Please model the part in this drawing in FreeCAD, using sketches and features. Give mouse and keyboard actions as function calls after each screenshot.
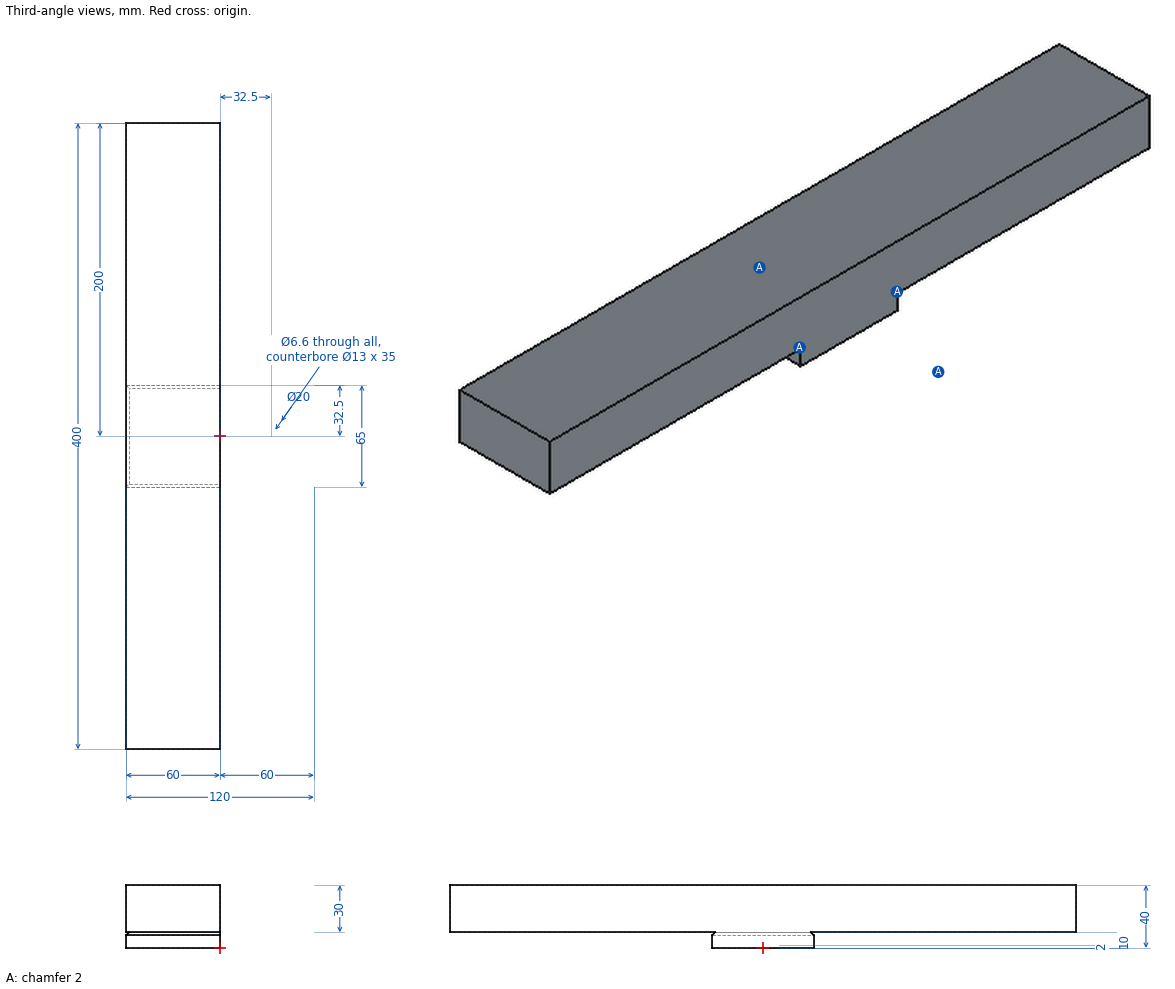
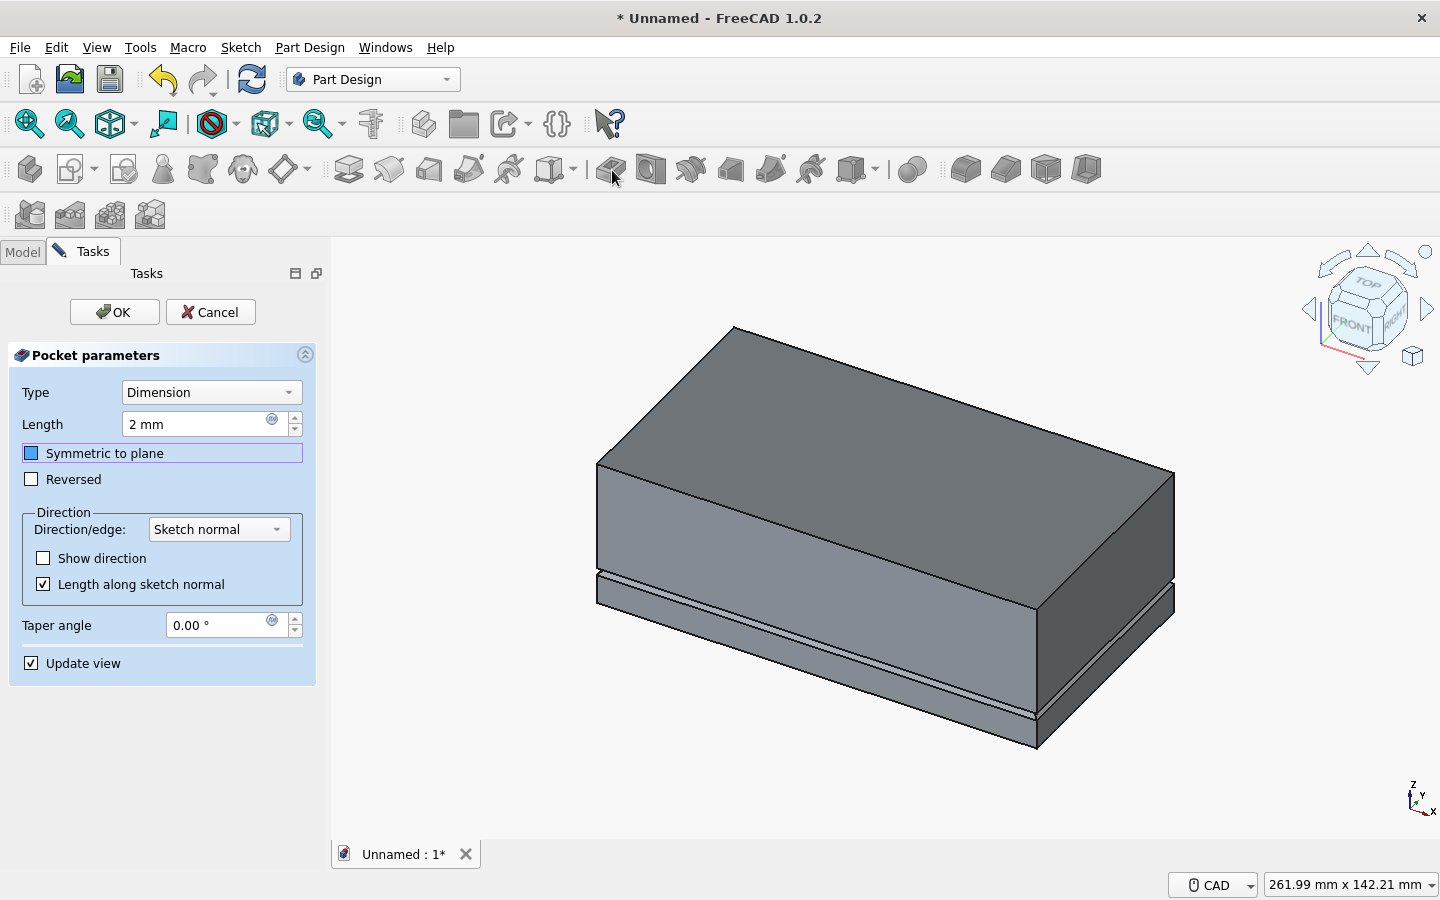
click(30, 479)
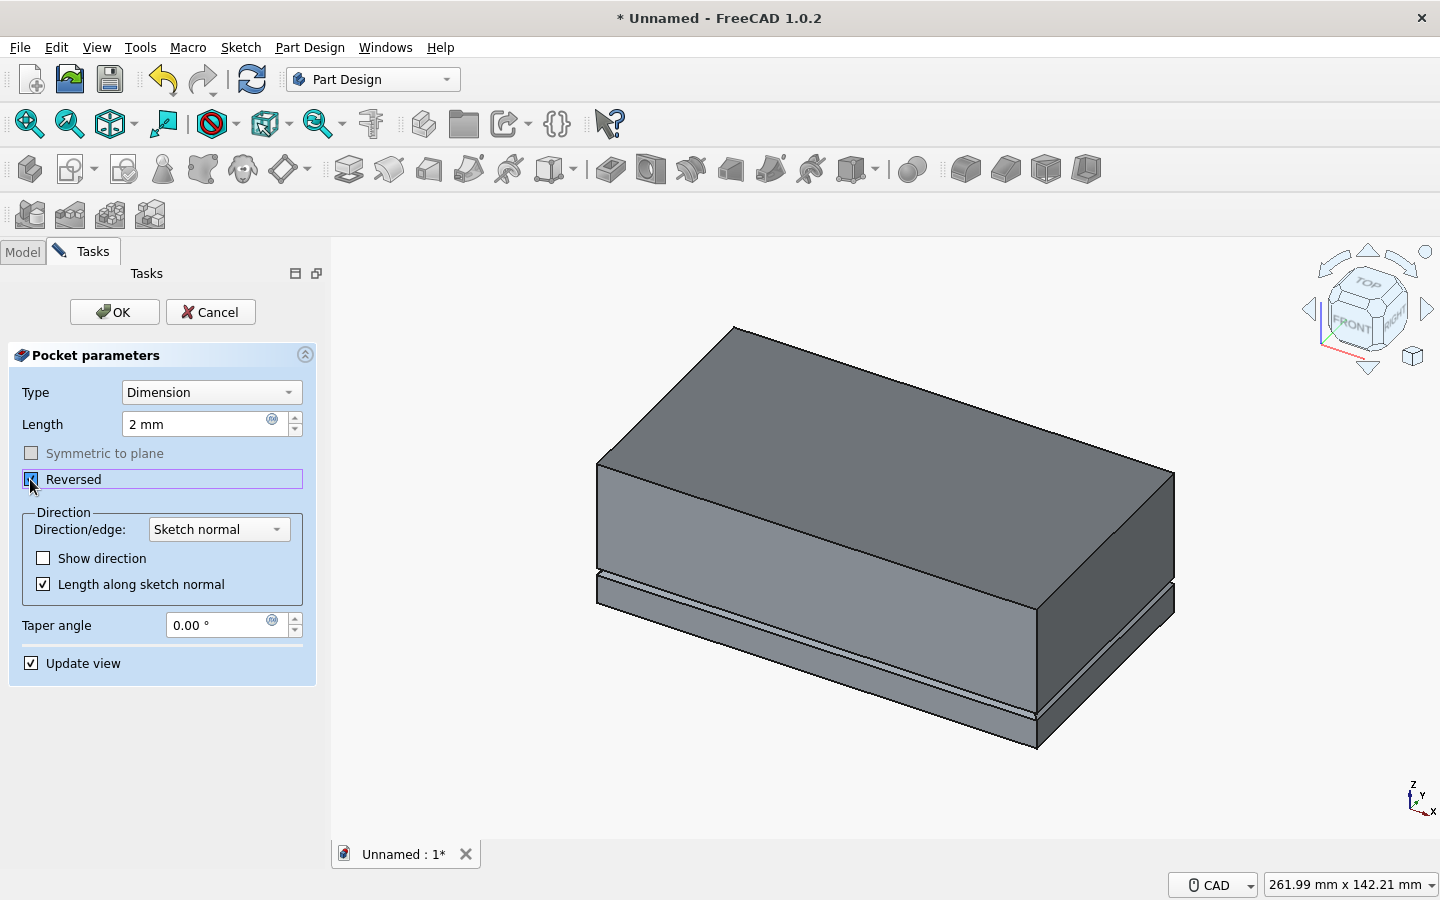
click(115, 312)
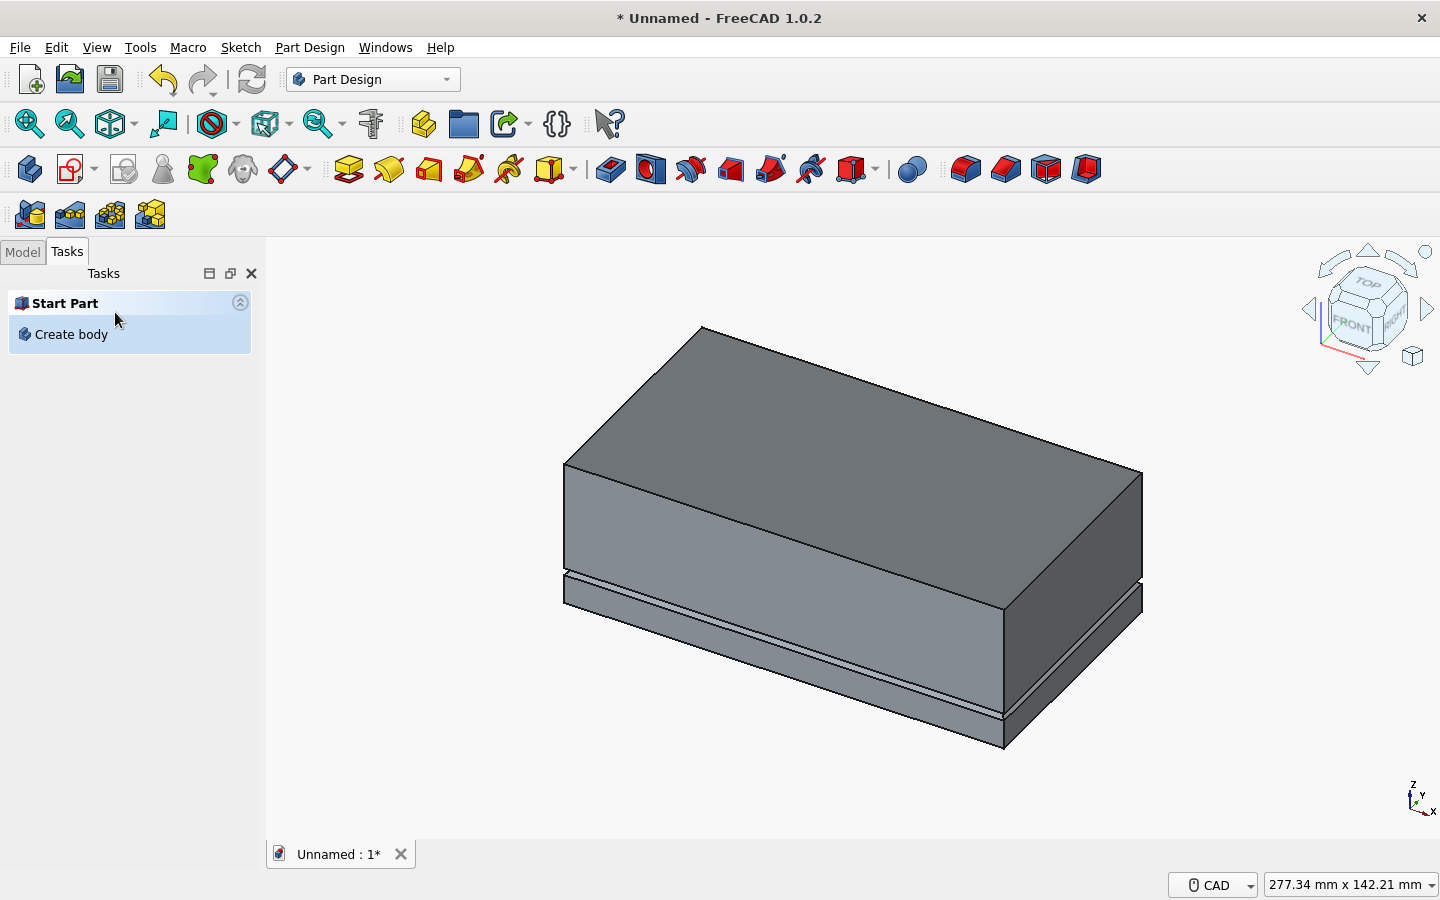
click(916, 488)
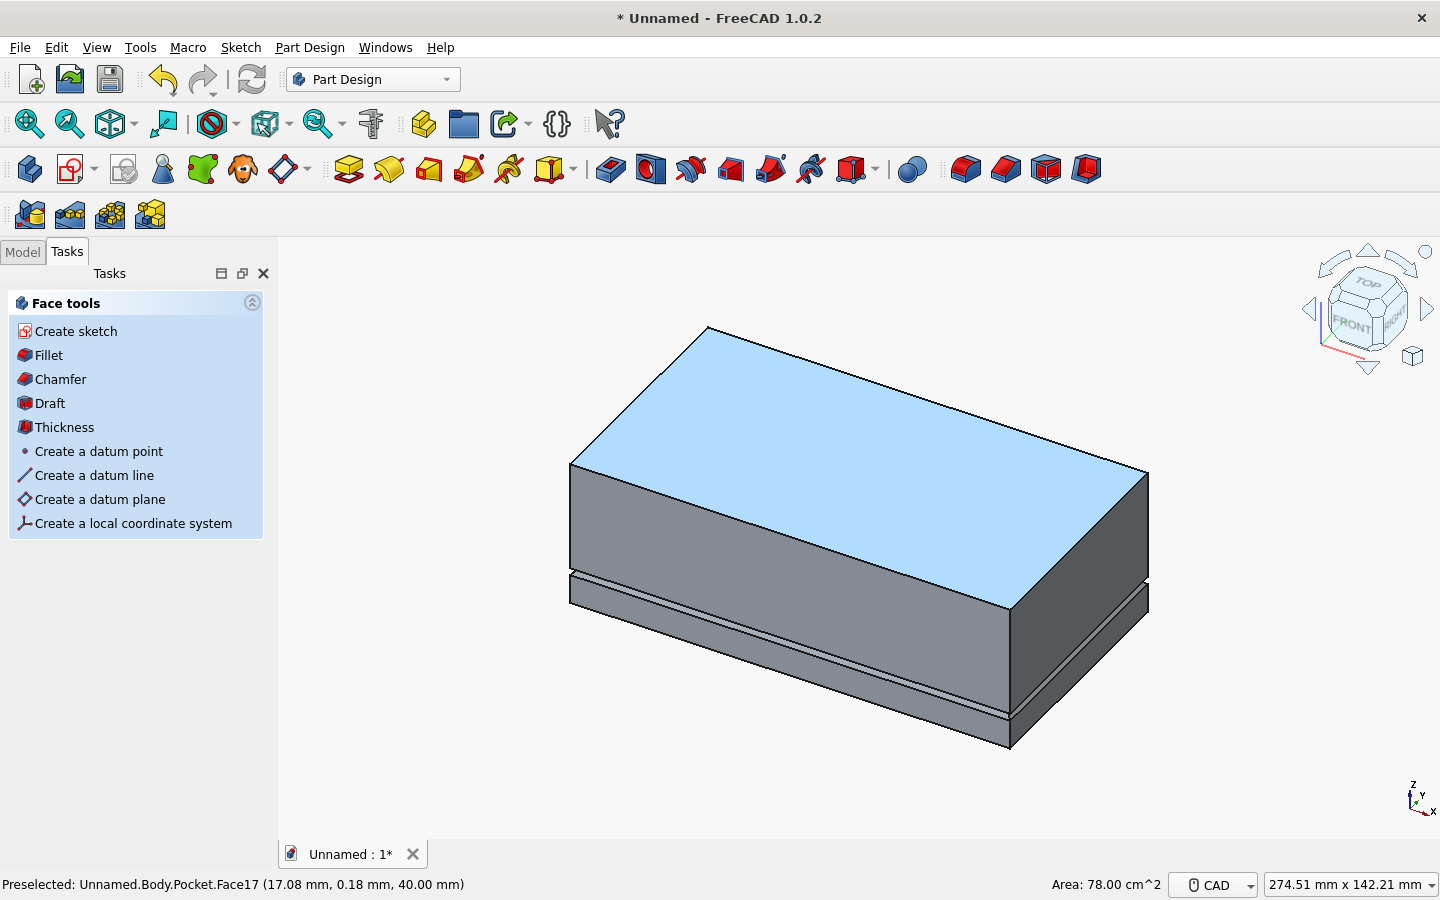
click(70, 170)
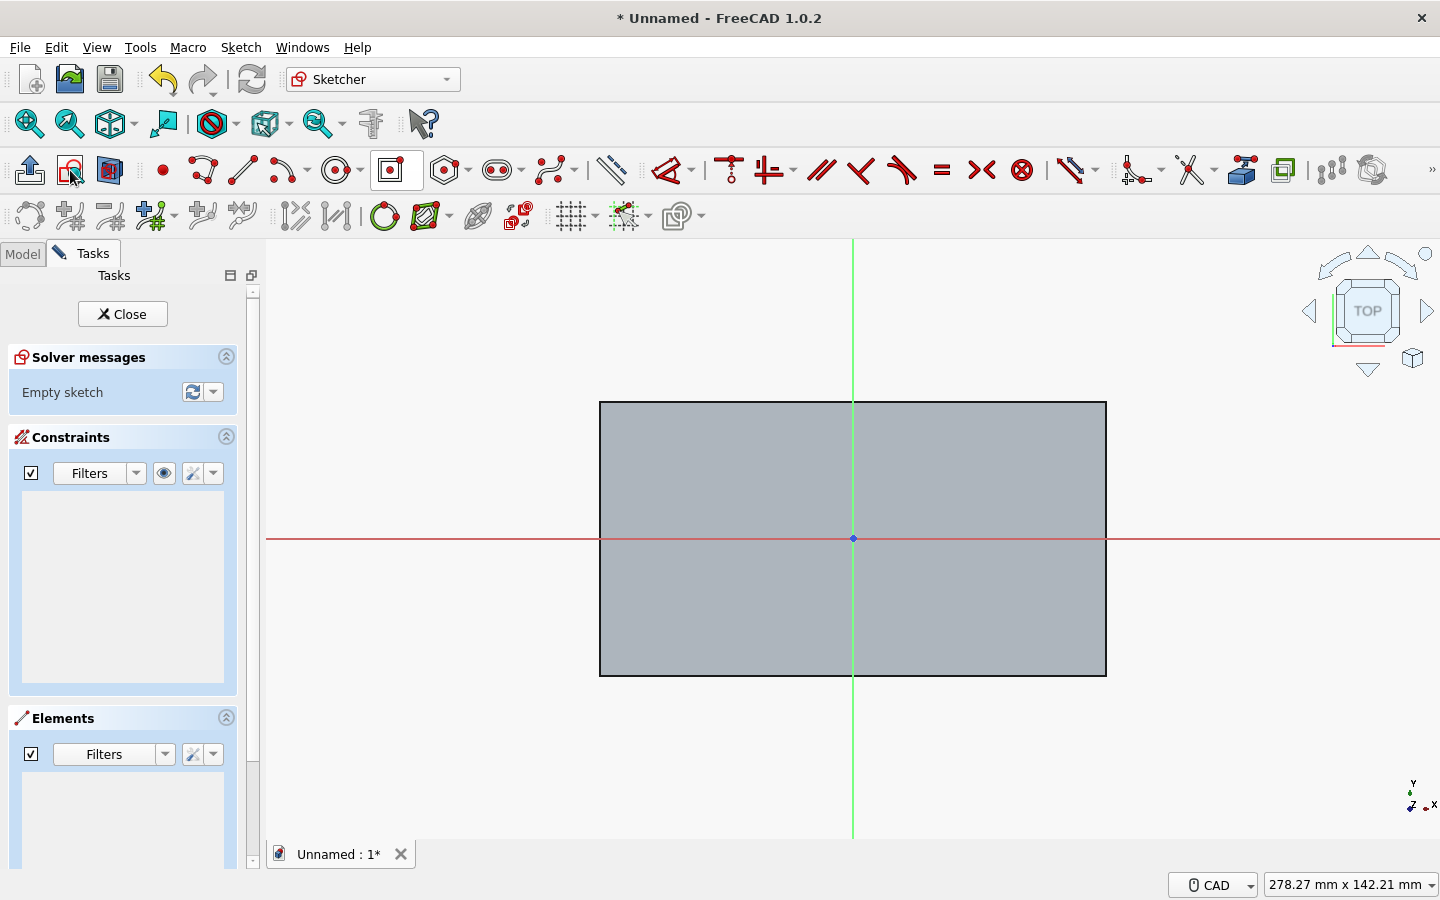
scroll(1007, 539, up, 13)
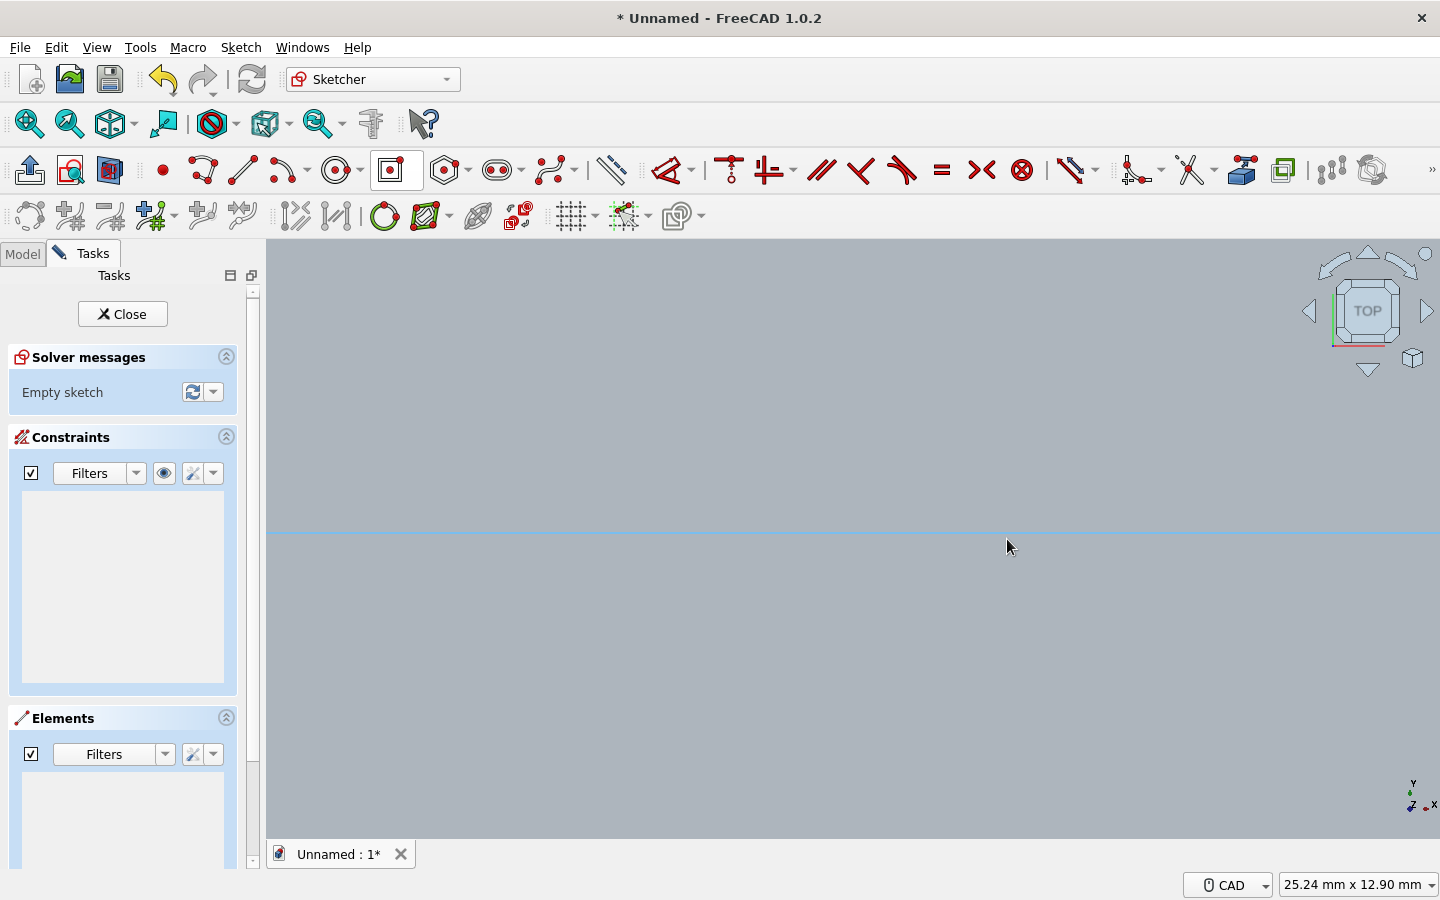
key(g)
key(c)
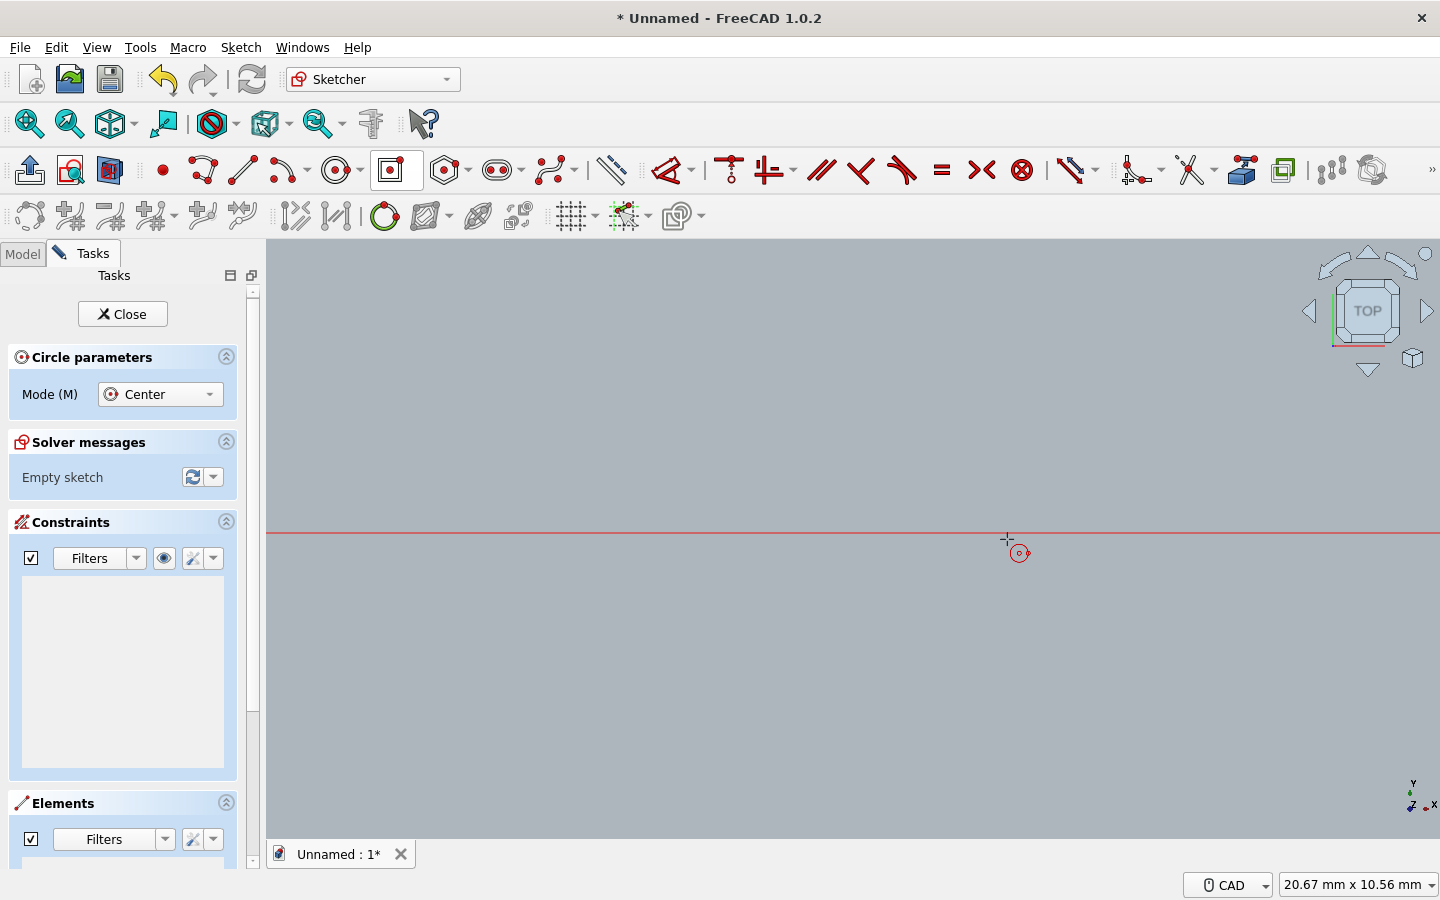
click(772, 533)
click(904, 400)
key(Escape)